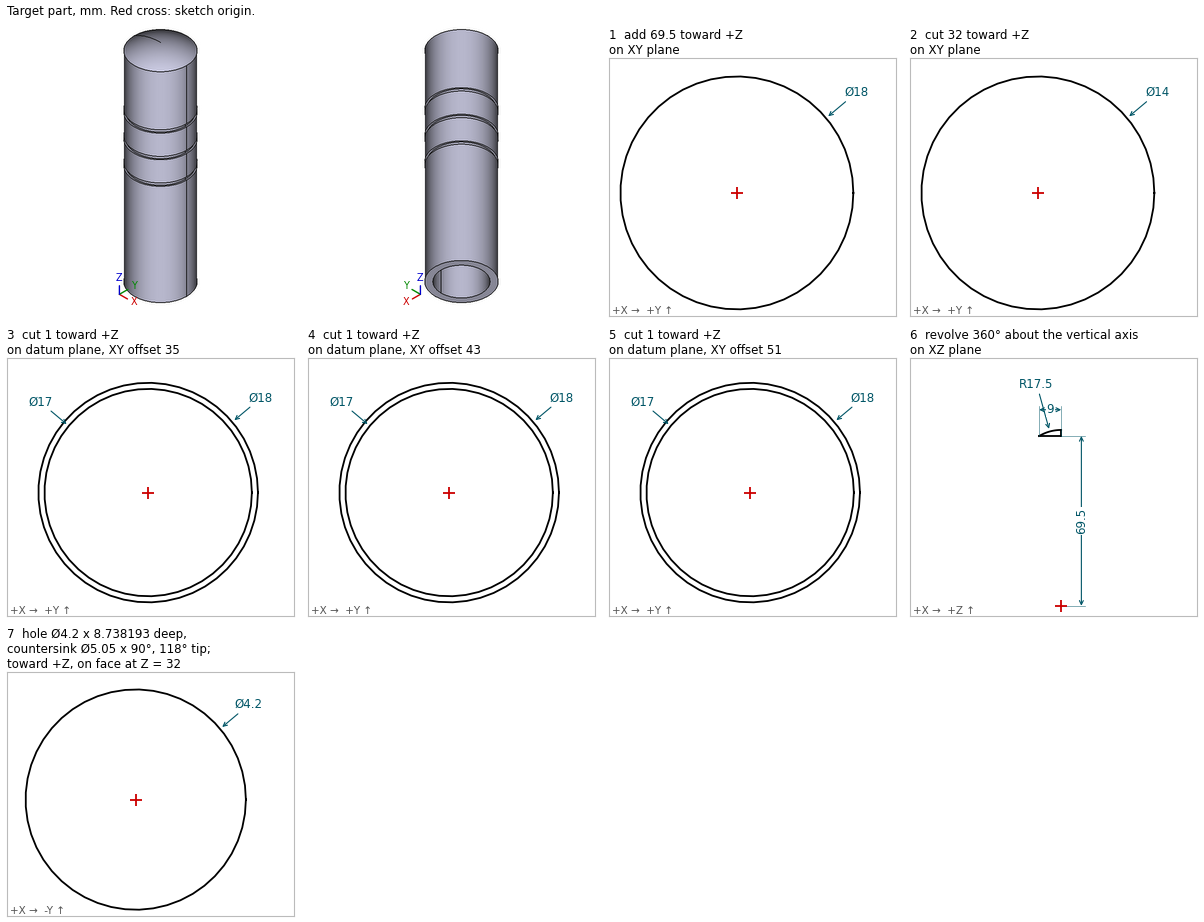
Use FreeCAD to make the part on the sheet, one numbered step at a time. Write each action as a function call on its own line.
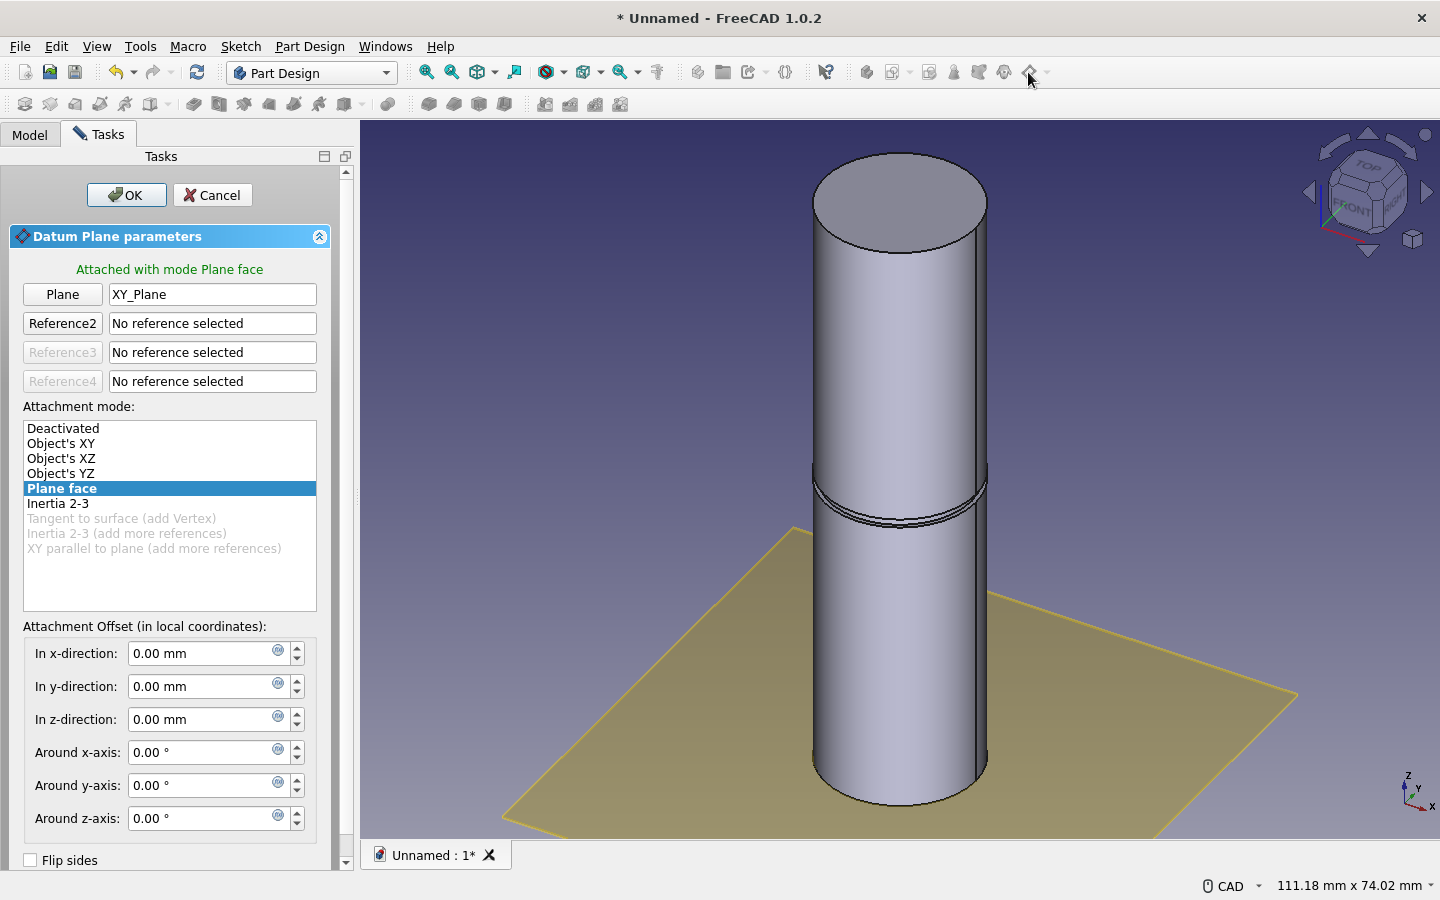
triple_click(210, 720)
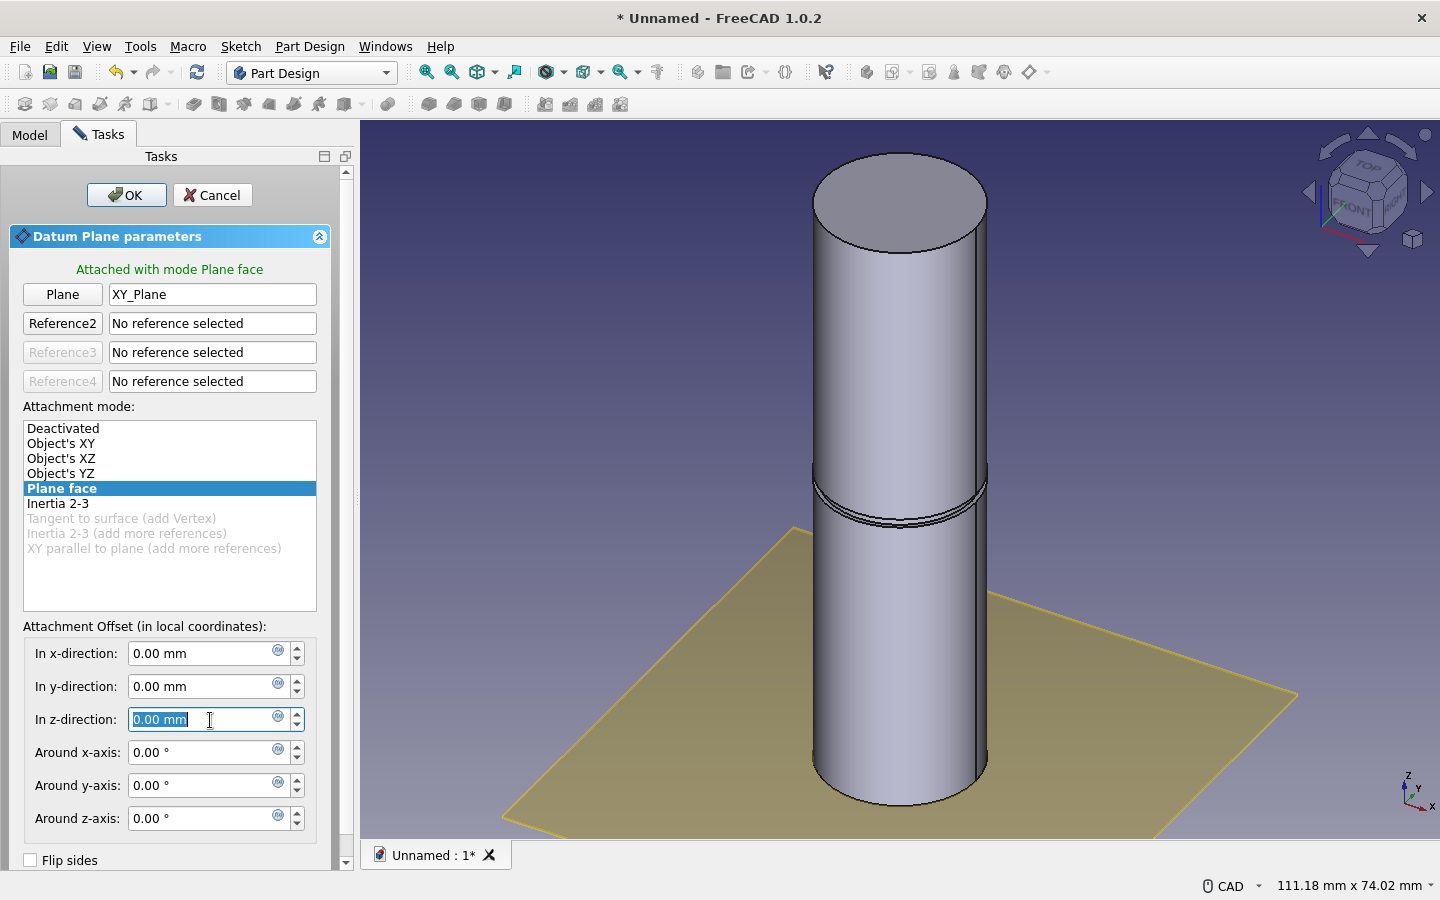
text(43)
key(Tab)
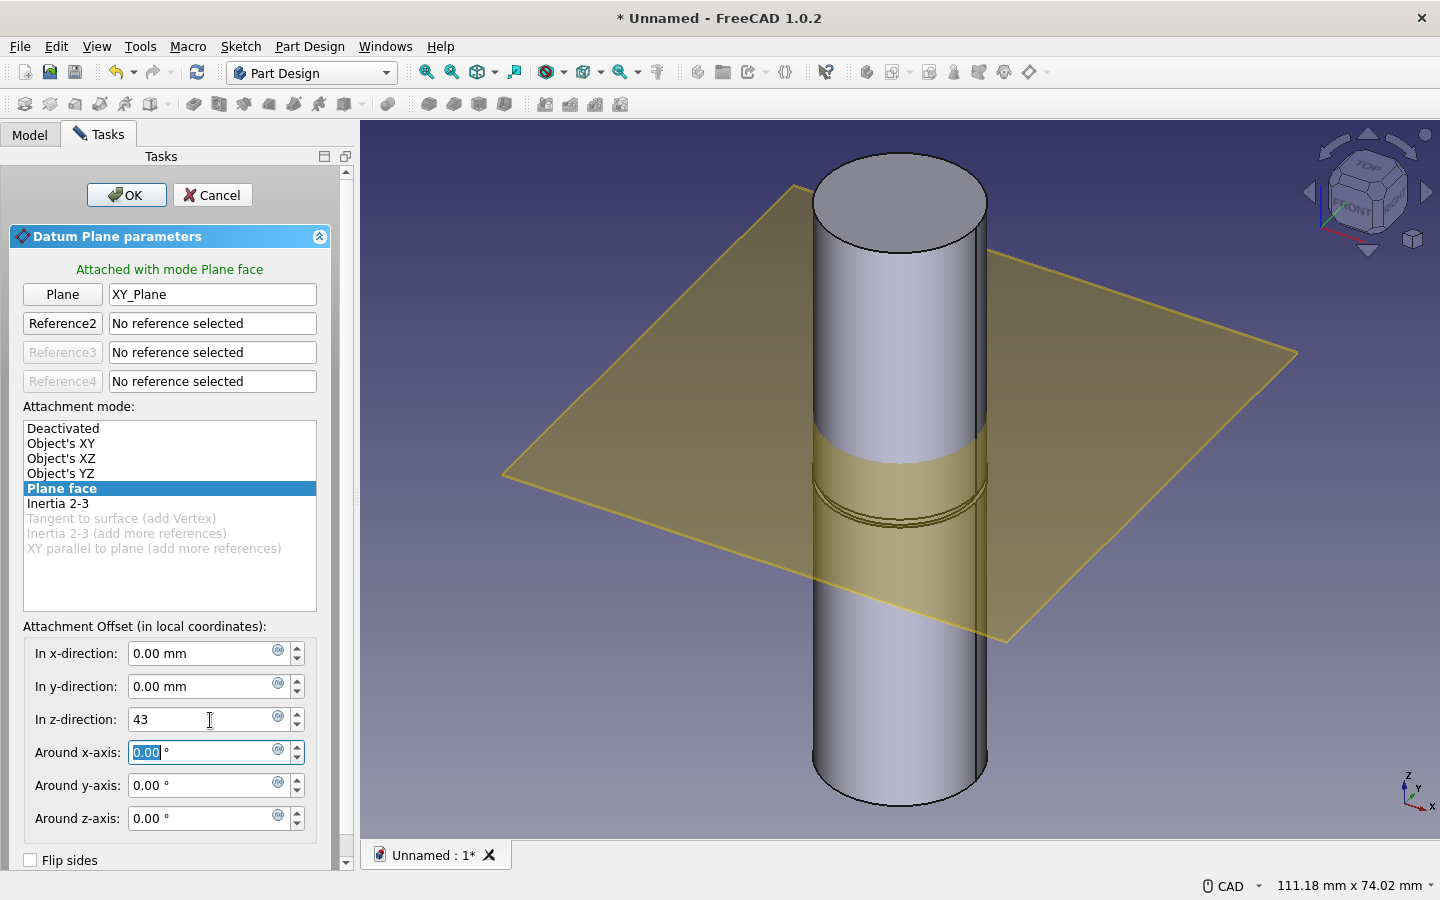
click(127, 195)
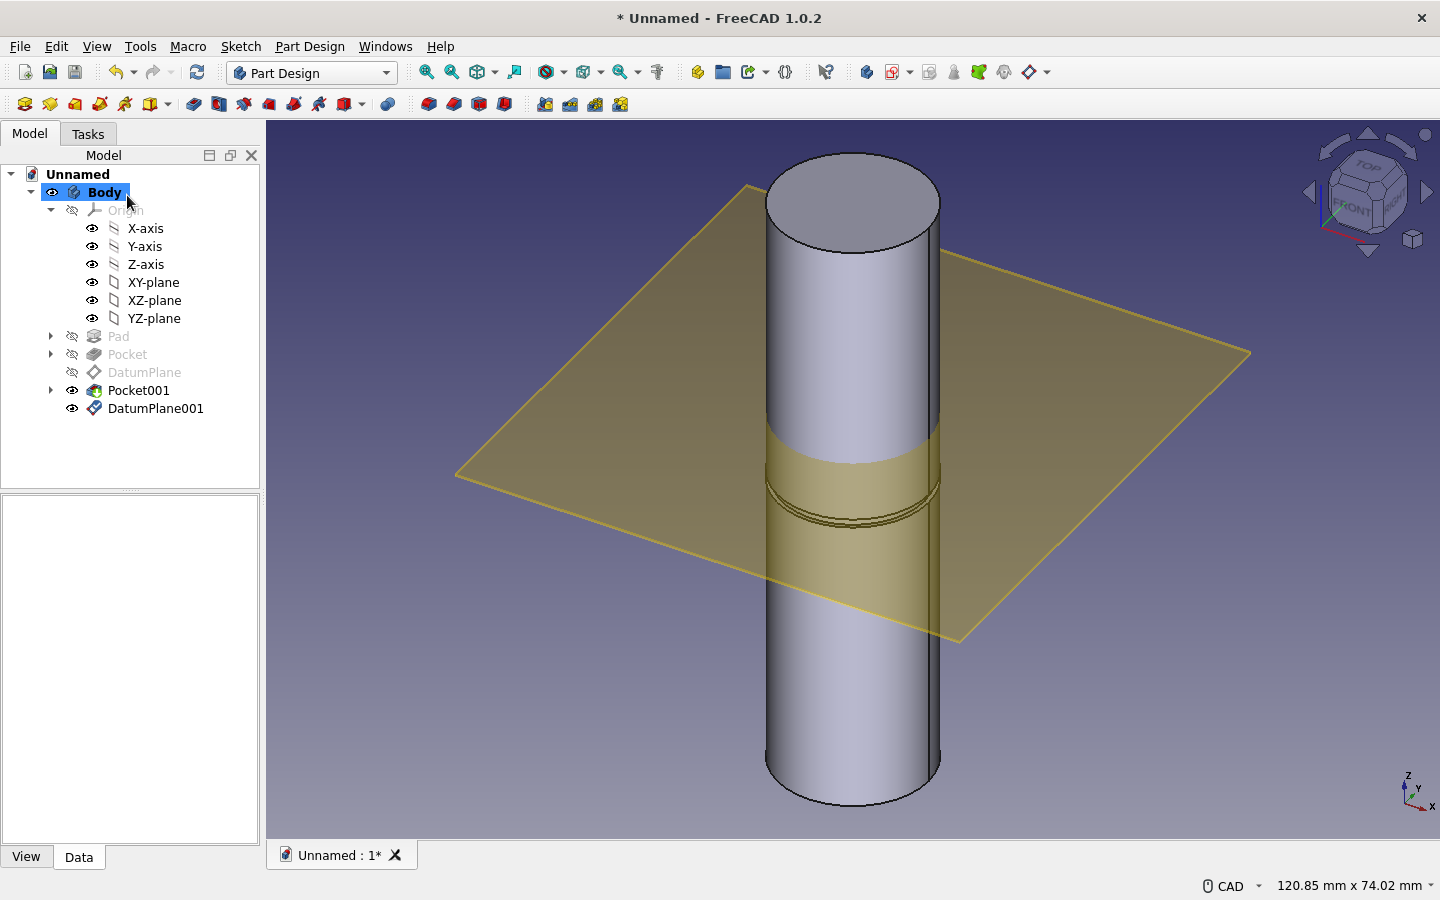
click(117, 408)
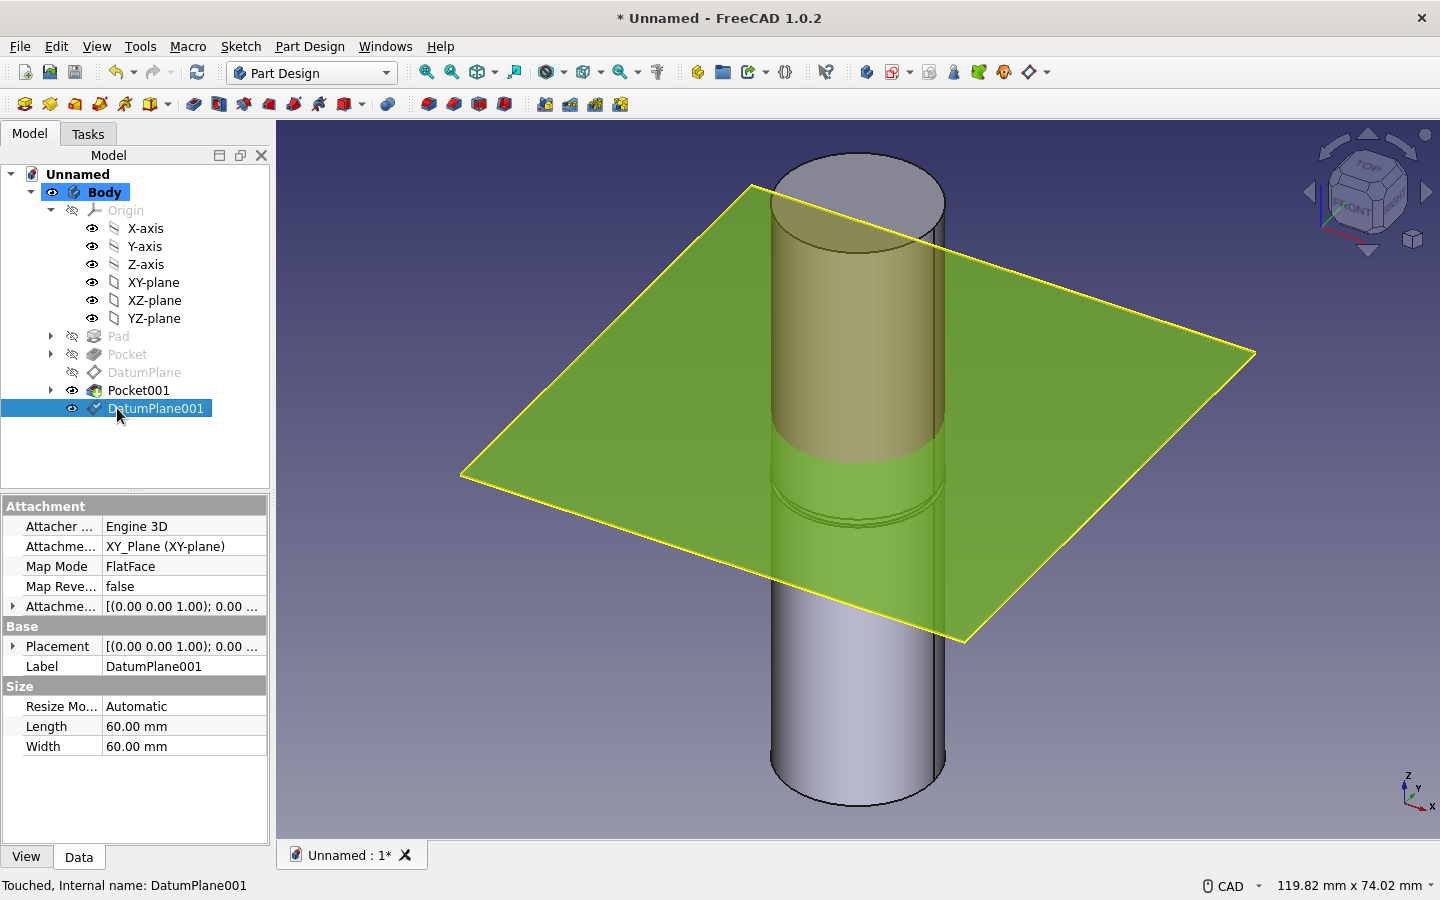
click(892, 72)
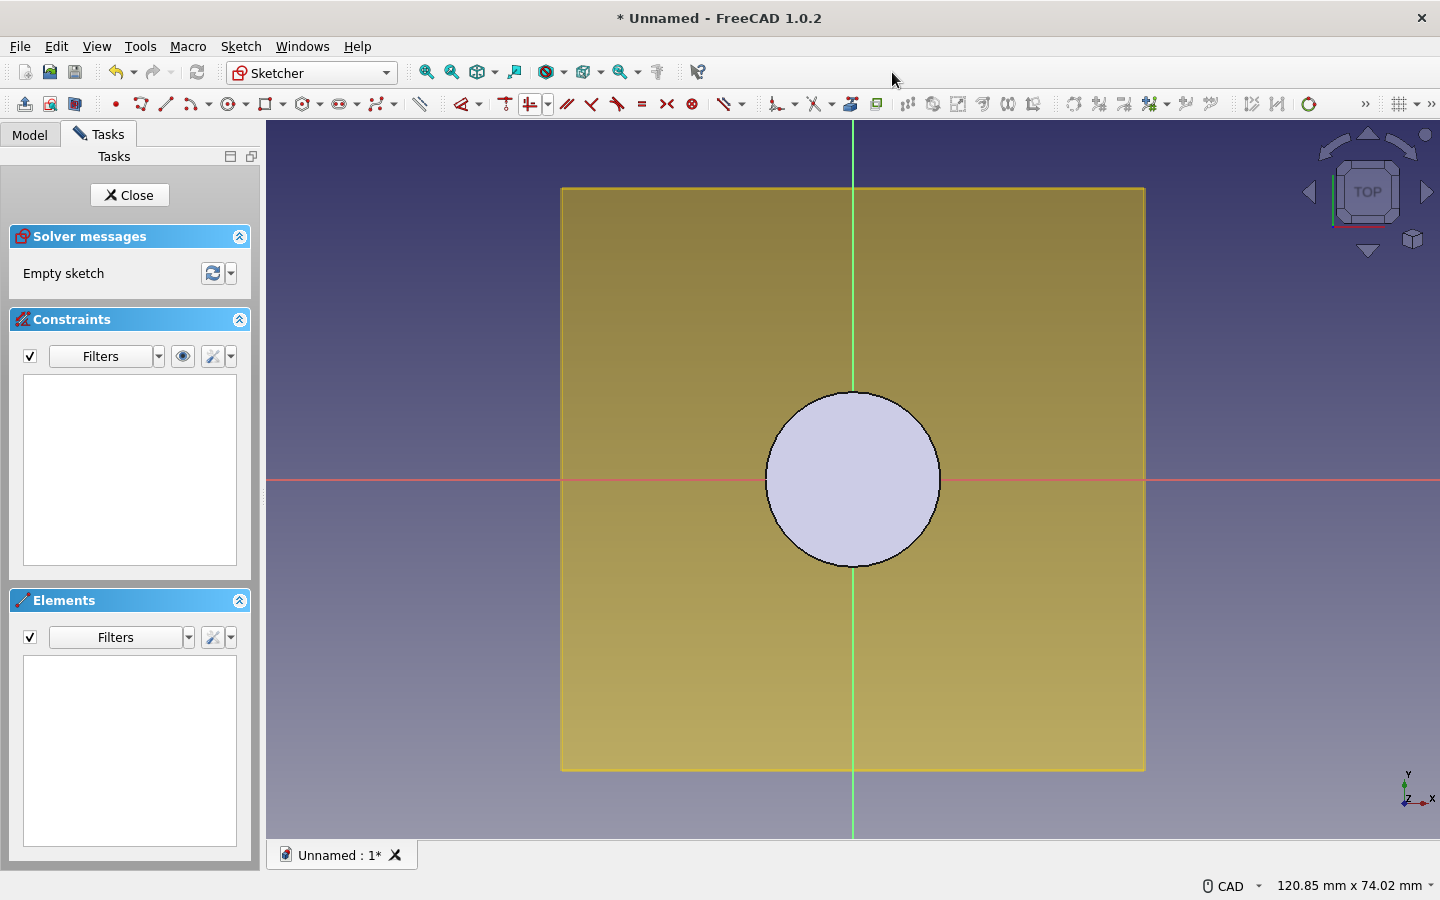
key(q)
key(s)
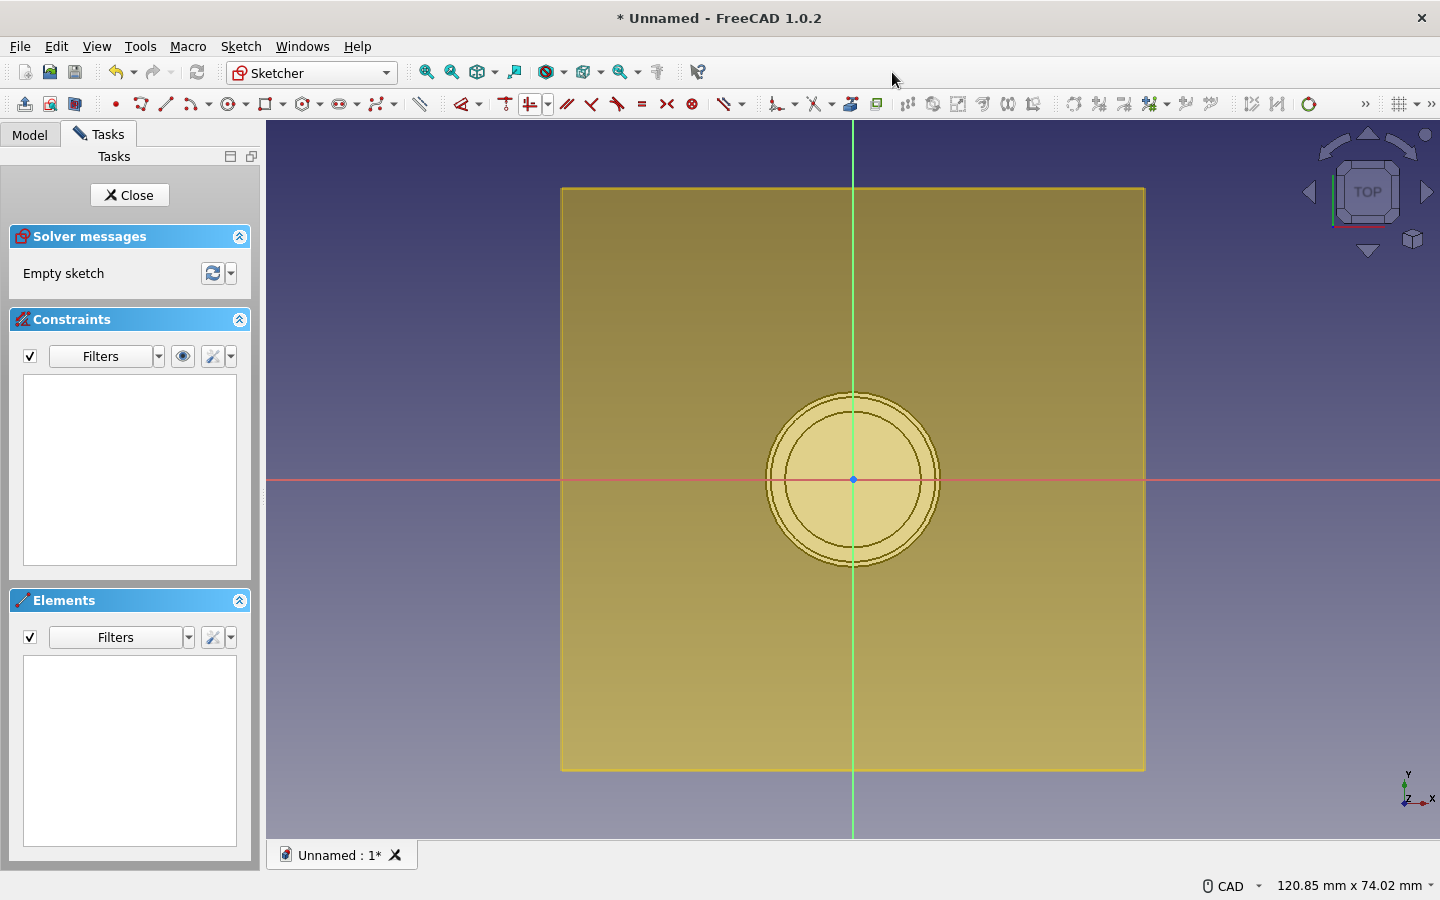
scroll(893, 480, up, 5)